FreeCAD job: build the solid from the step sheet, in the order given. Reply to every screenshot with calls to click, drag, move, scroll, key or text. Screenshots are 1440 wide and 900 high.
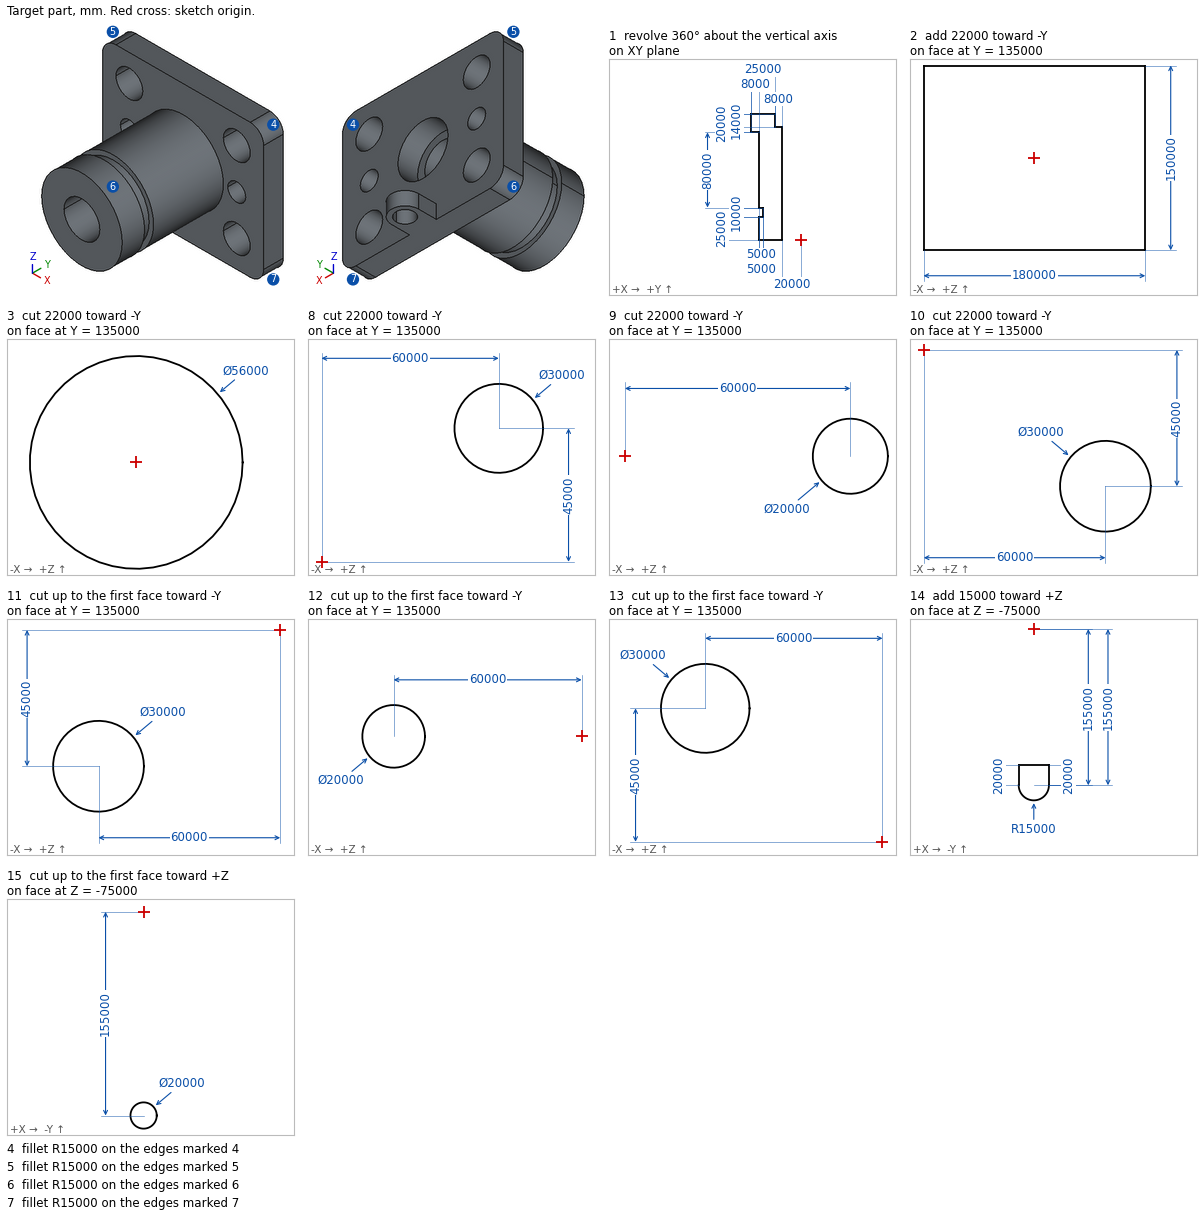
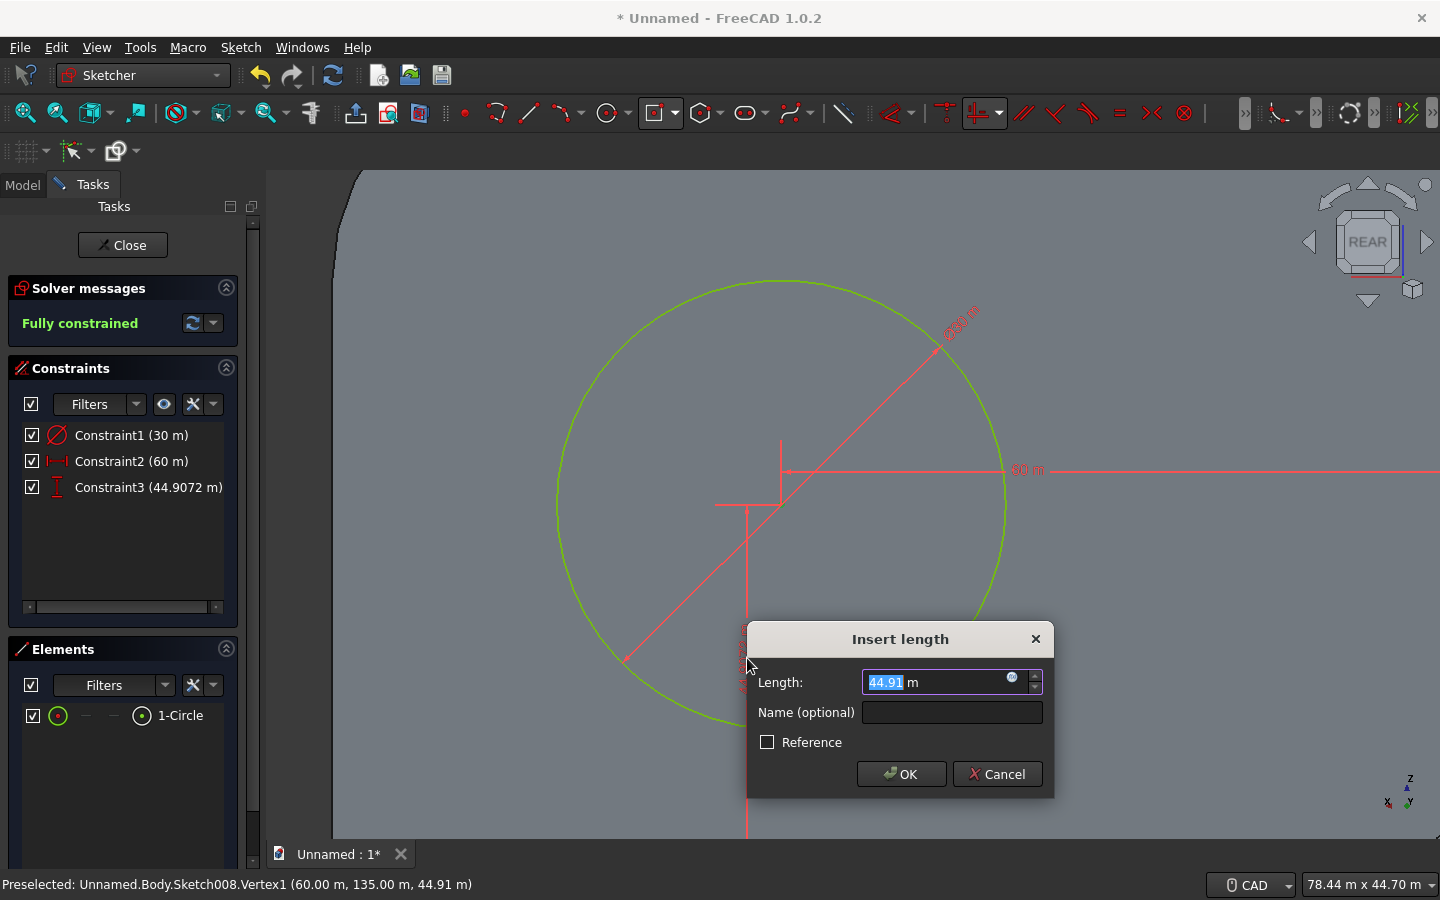
key(ctrl+a)
text(45000 mm)
key(Return)
key(Escape)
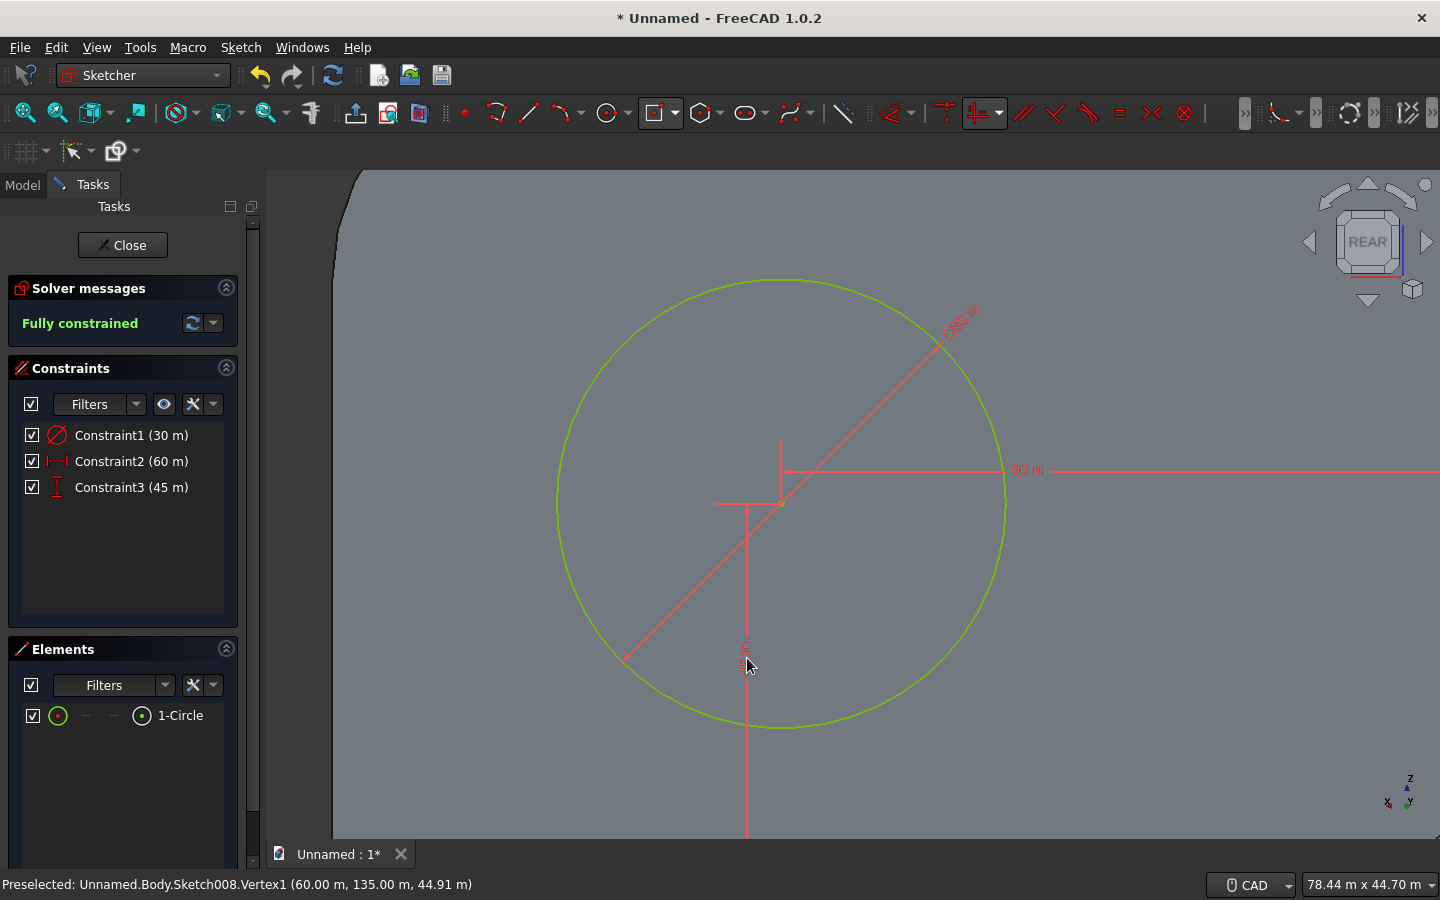
click(123, 245)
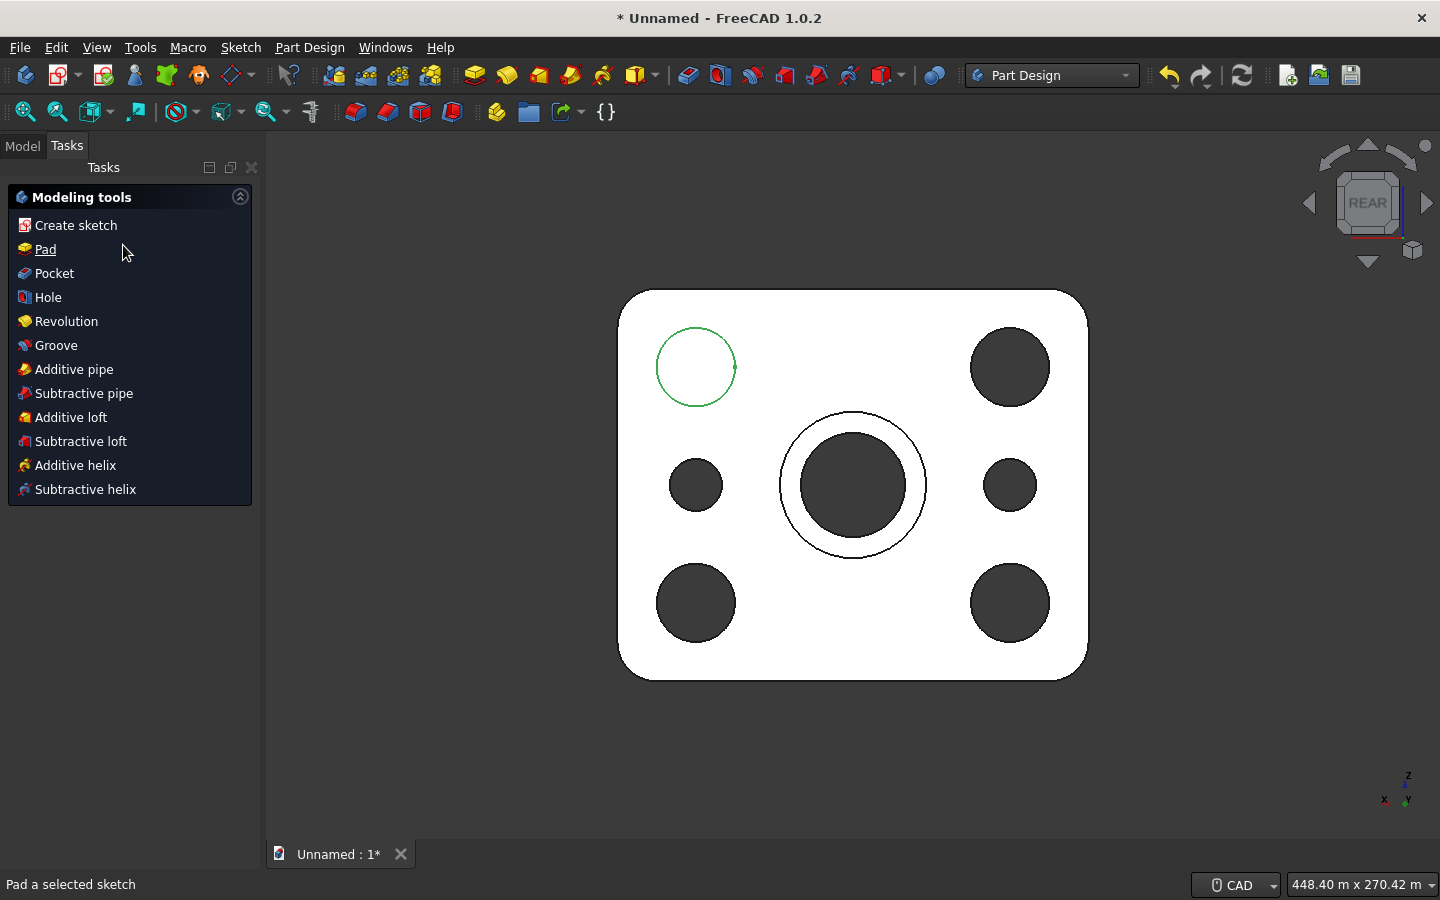
click(690, 76)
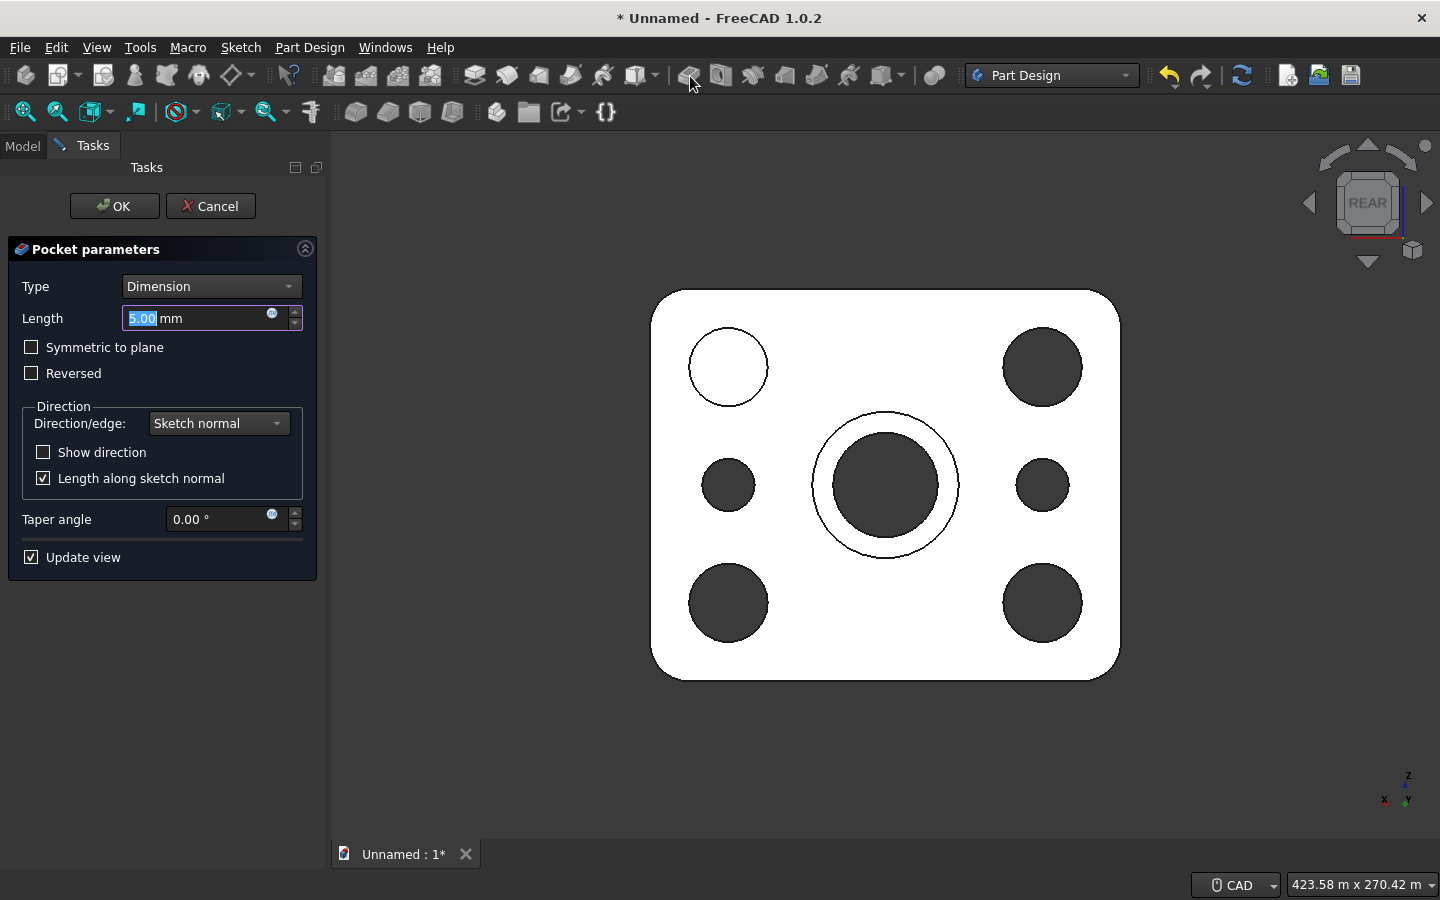
click(212, 286)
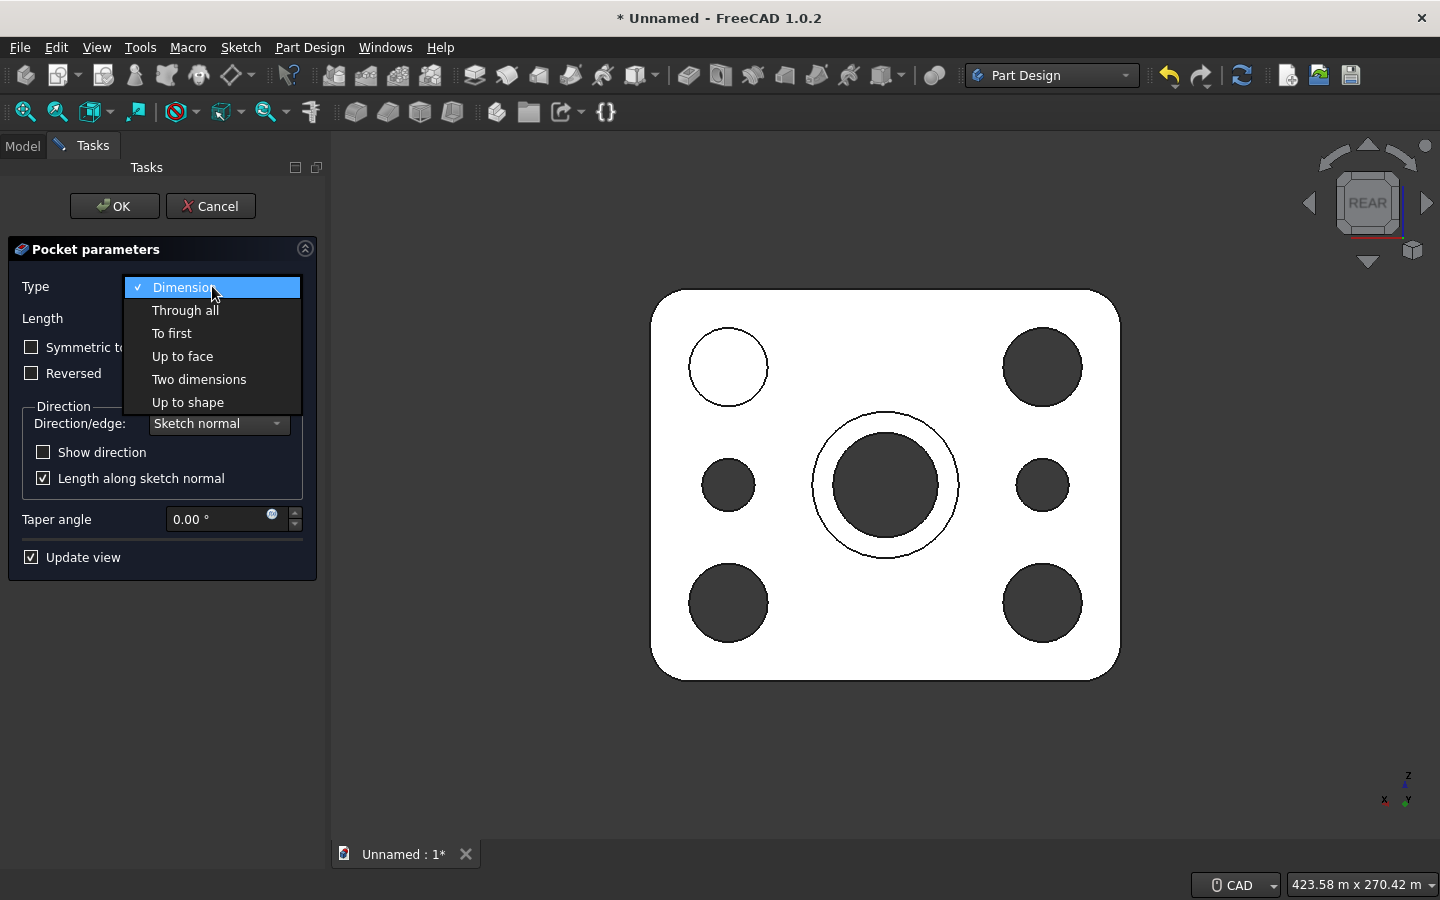
click(212, 334)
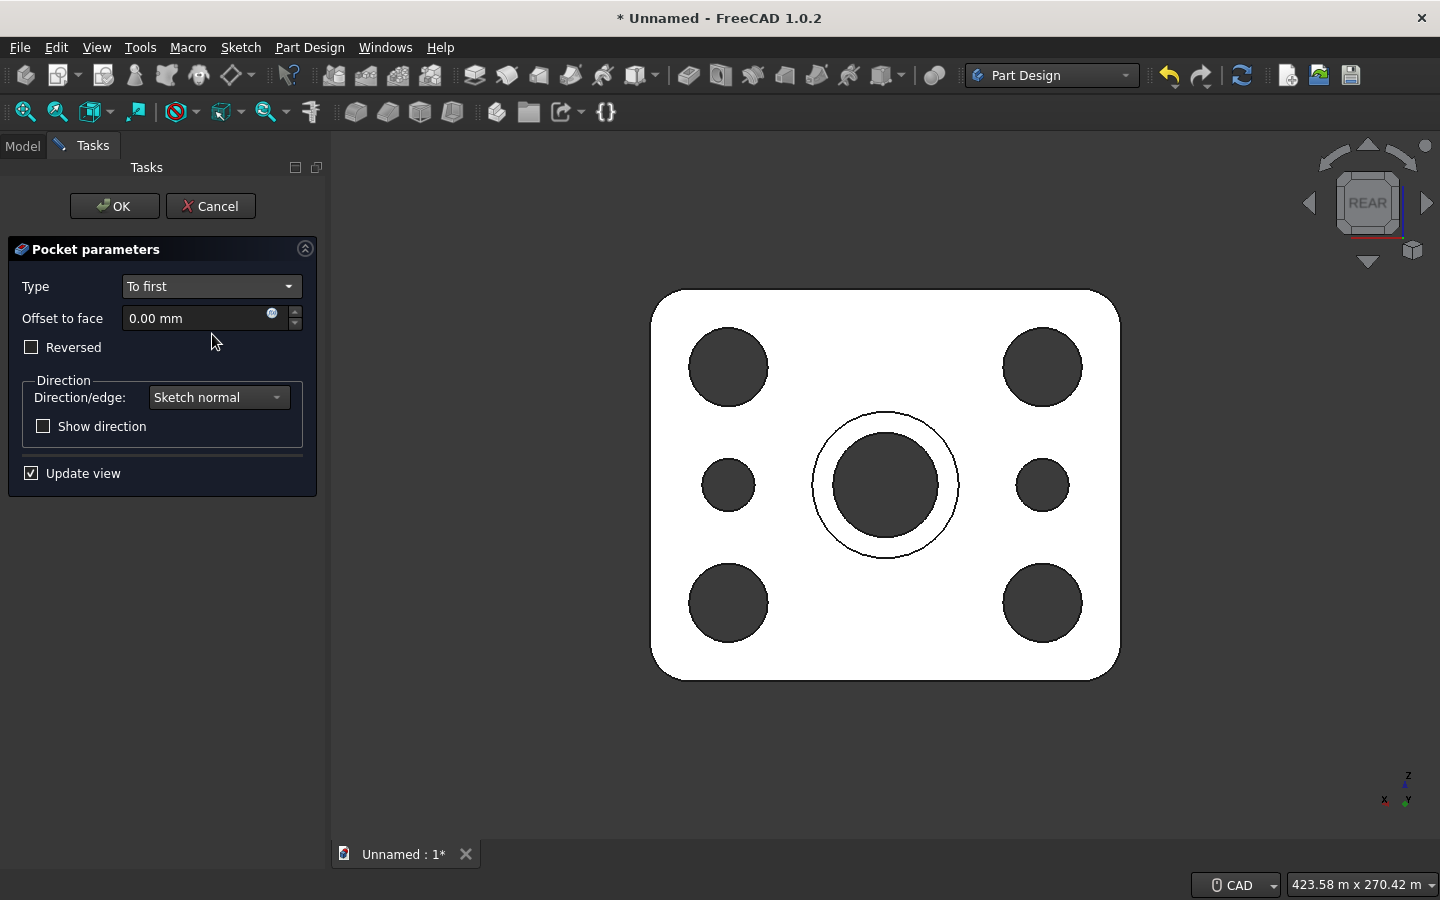
click(115, 206)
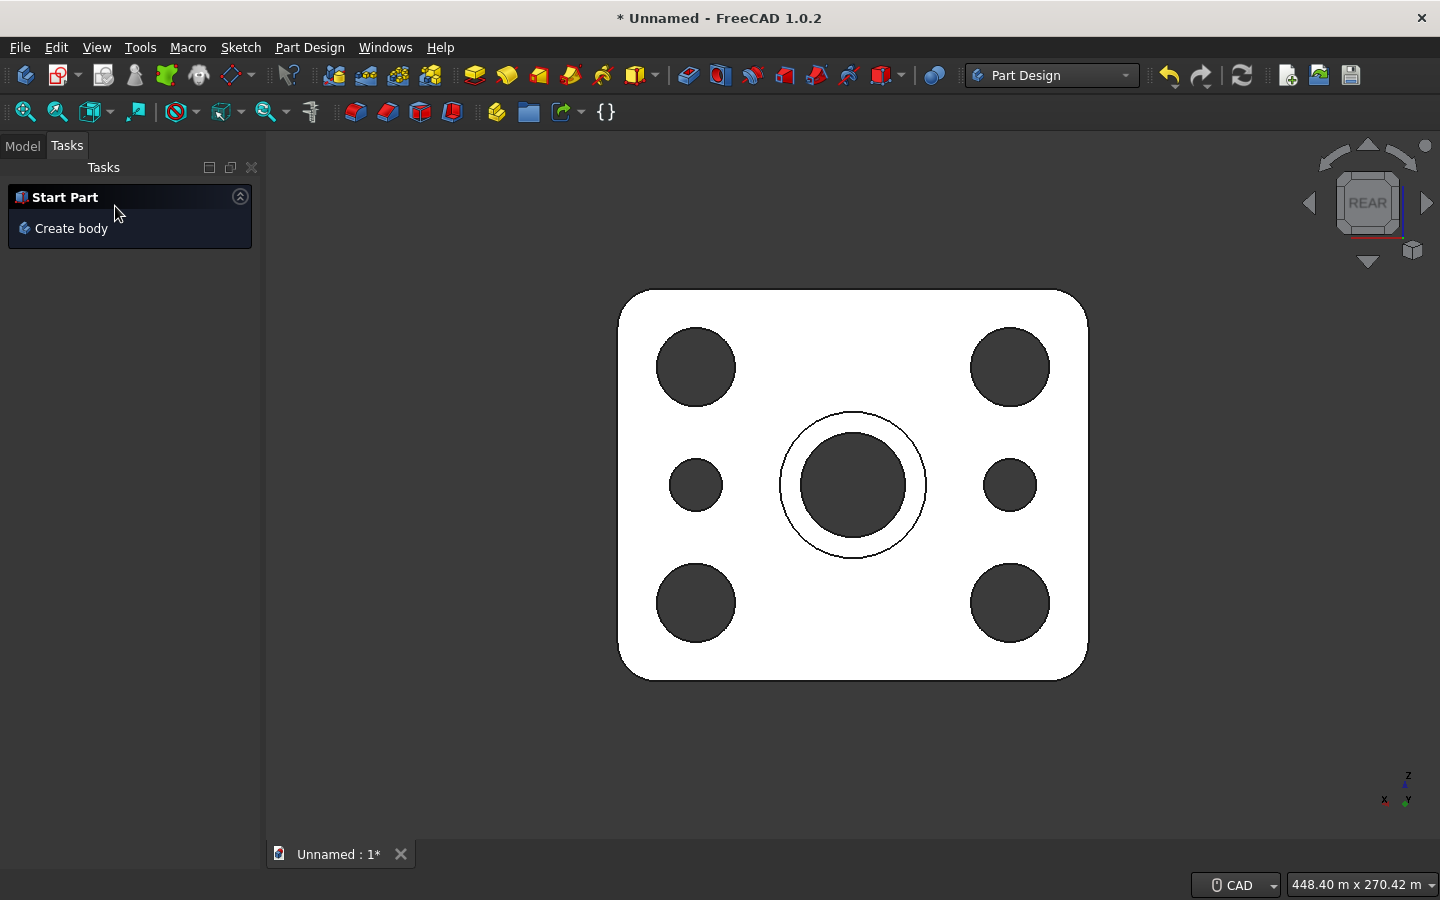
key(5)